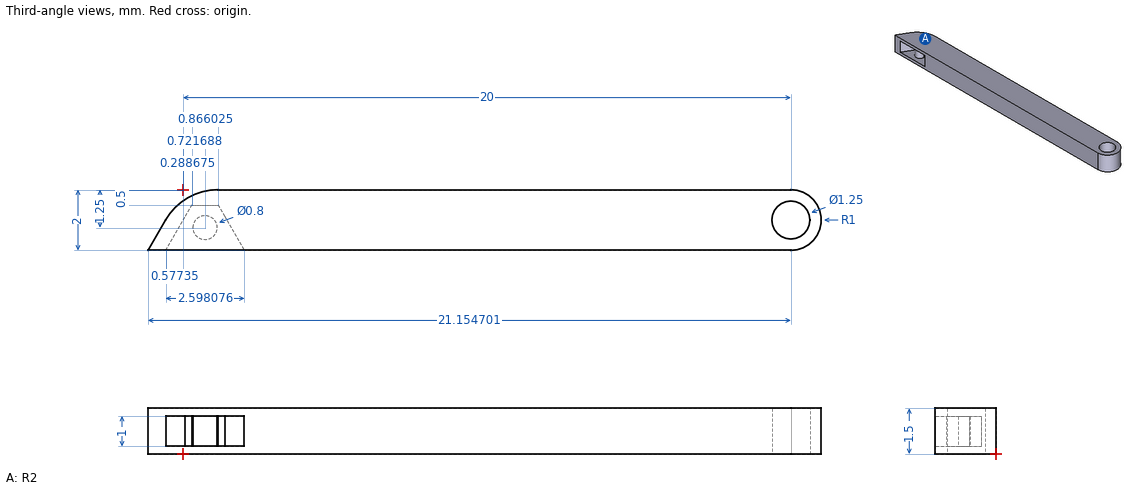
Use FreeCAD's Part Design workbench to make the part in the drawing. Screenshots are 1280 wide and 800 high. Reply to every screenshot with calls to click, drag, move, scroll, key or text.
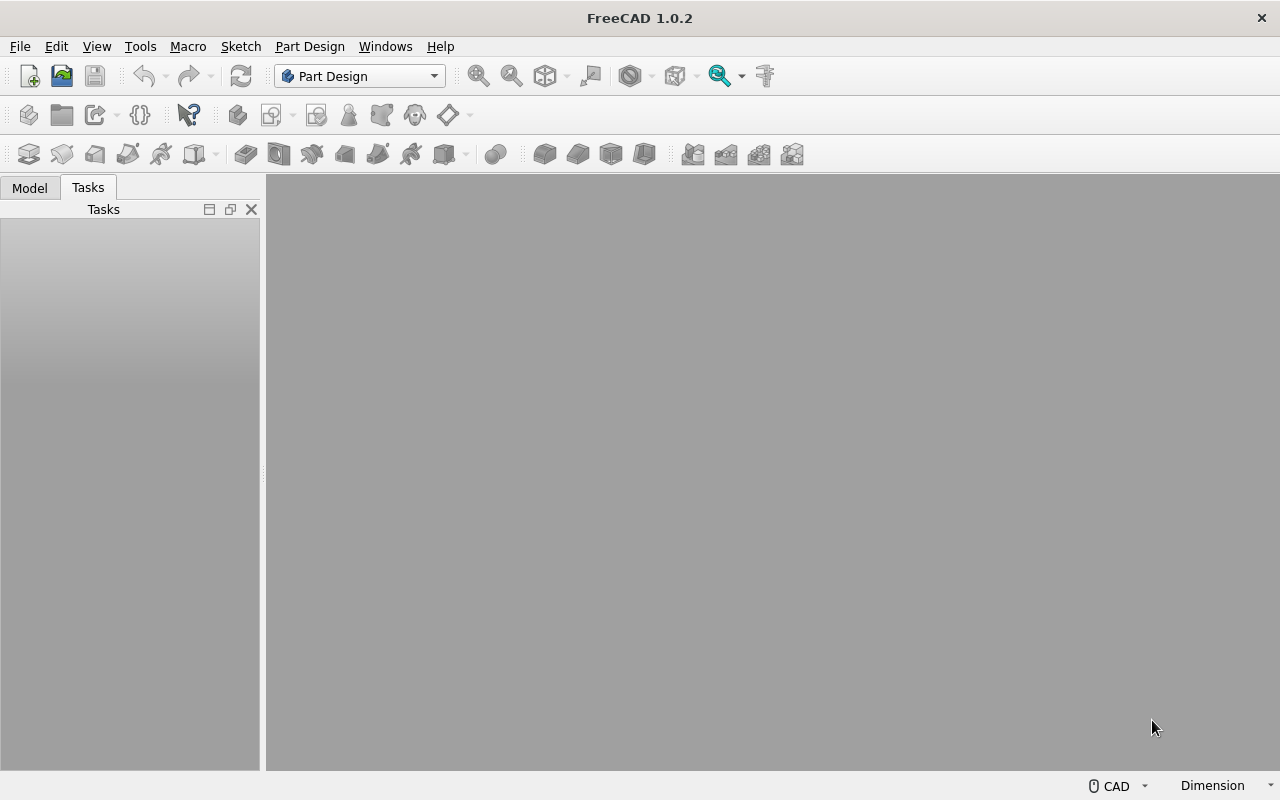
key(ctrl+n)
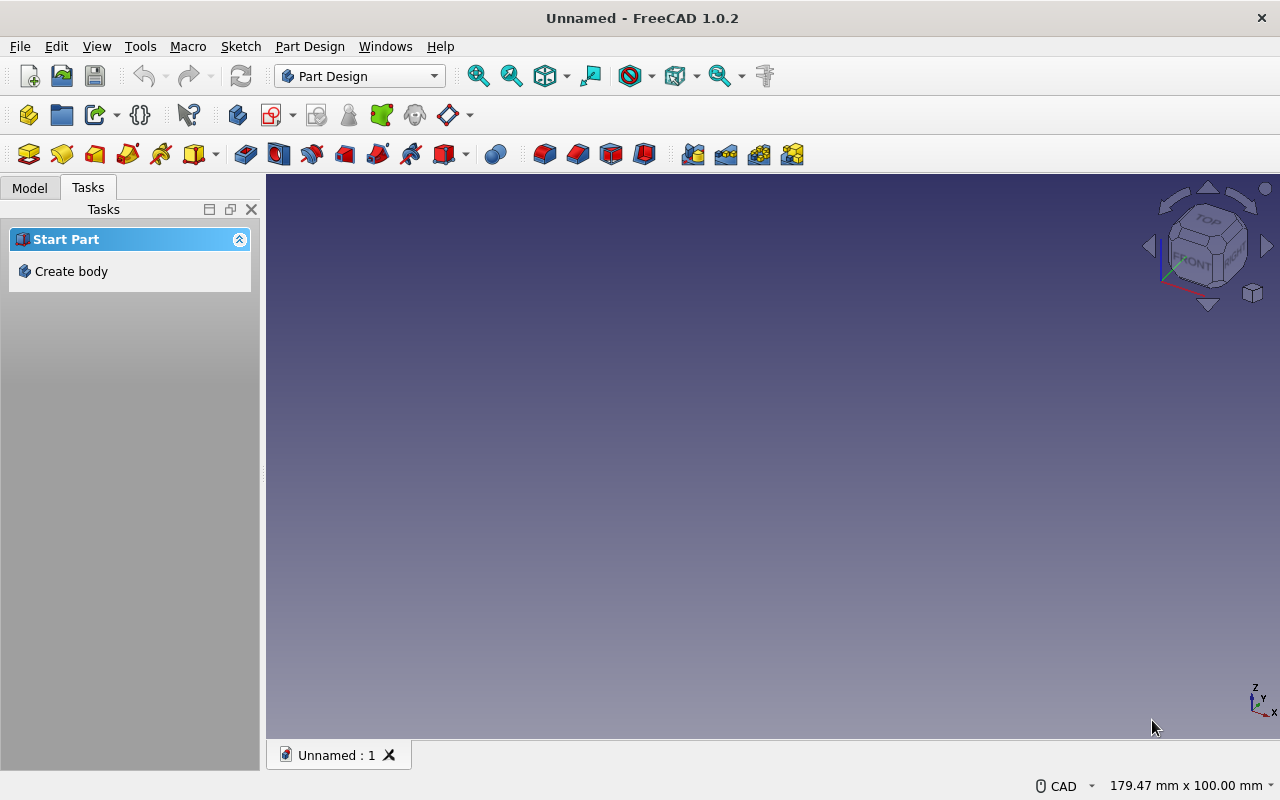
click(270, 116)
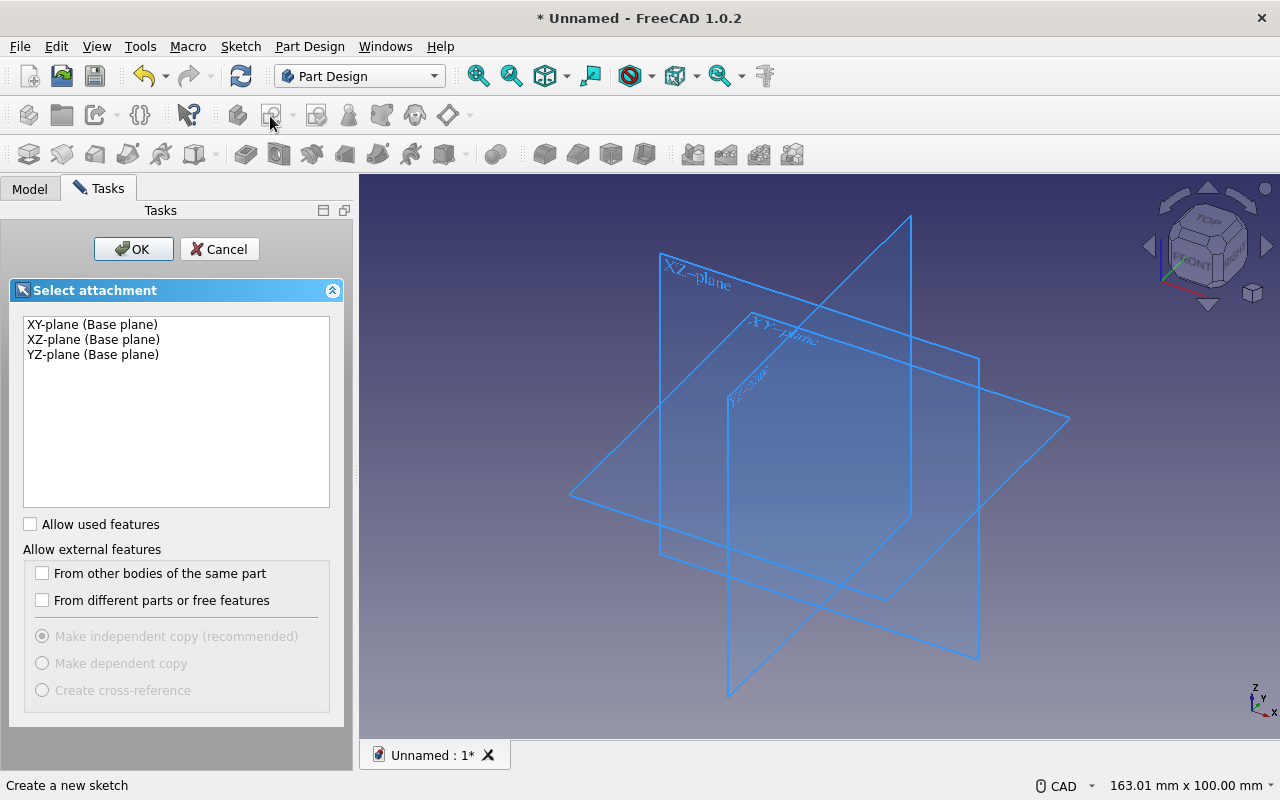
click(84, 324)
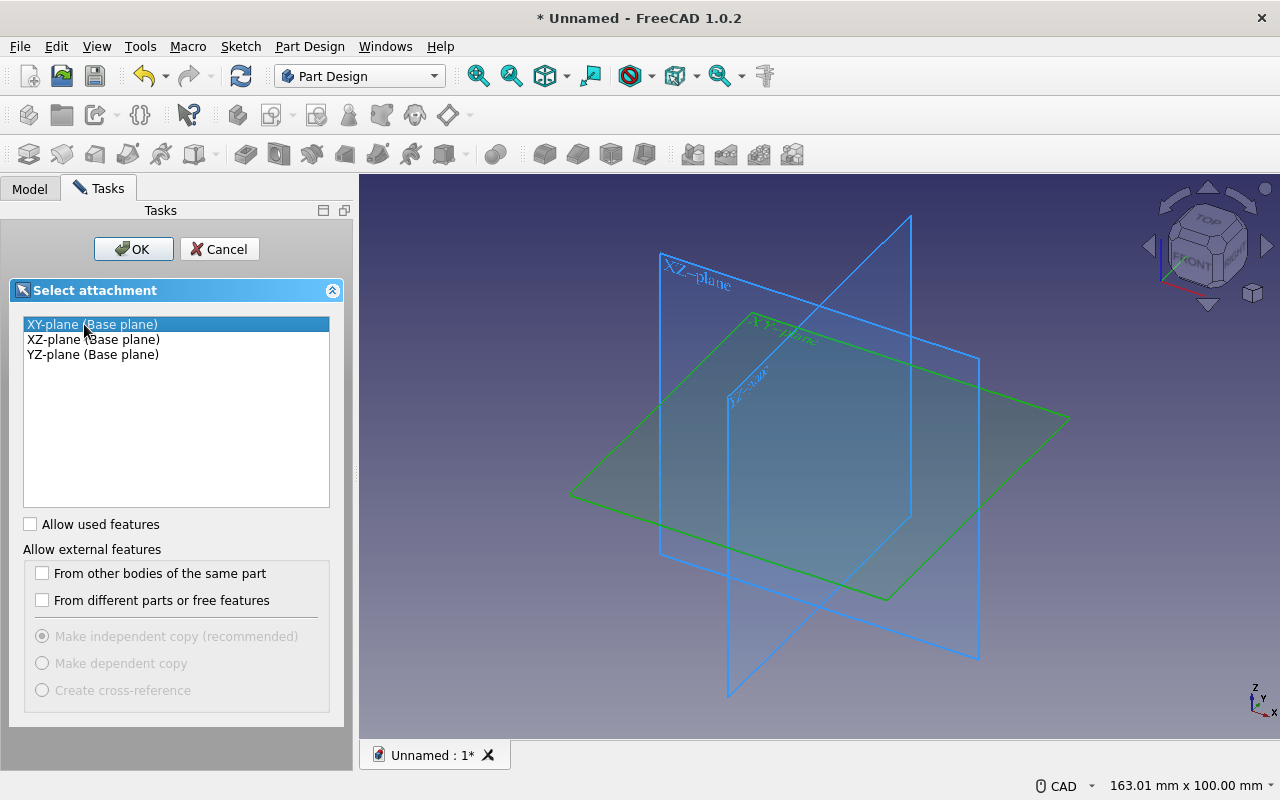
click(134, 249)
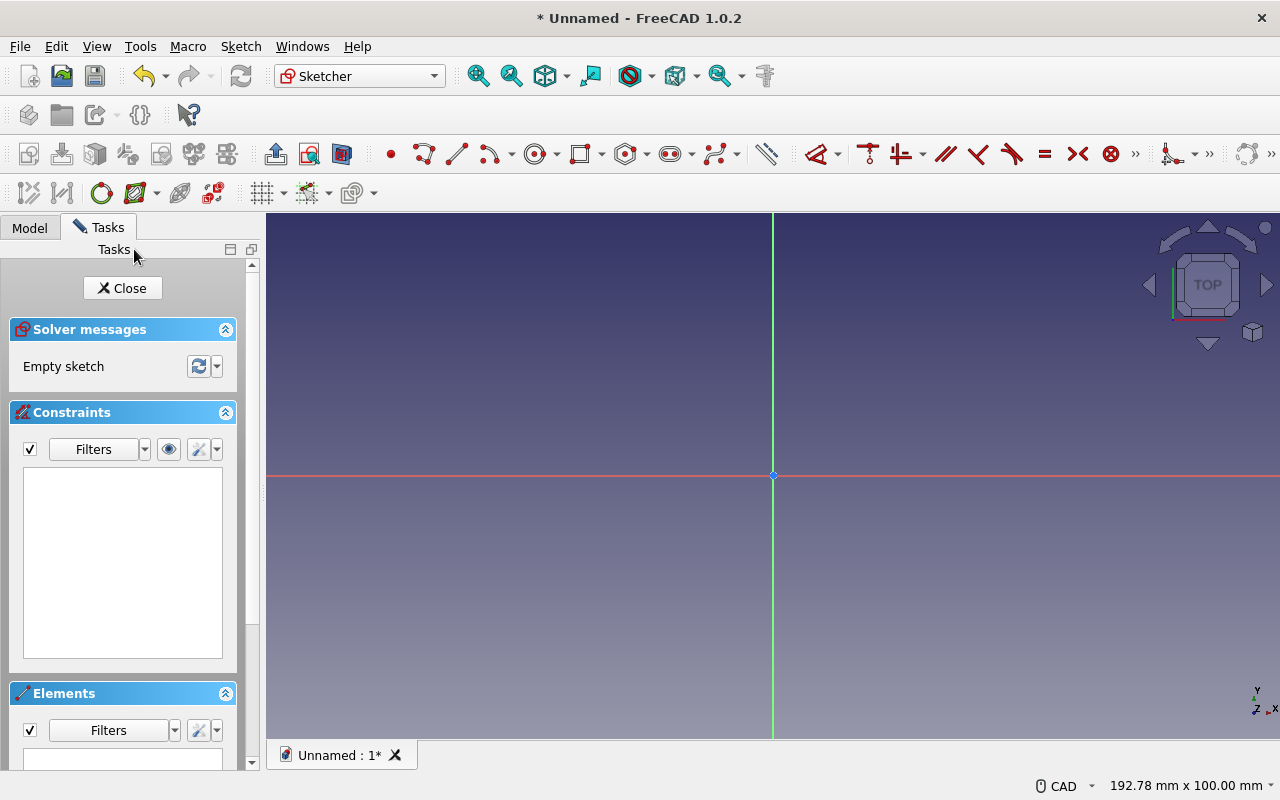
scroll(856, 483, up, 8)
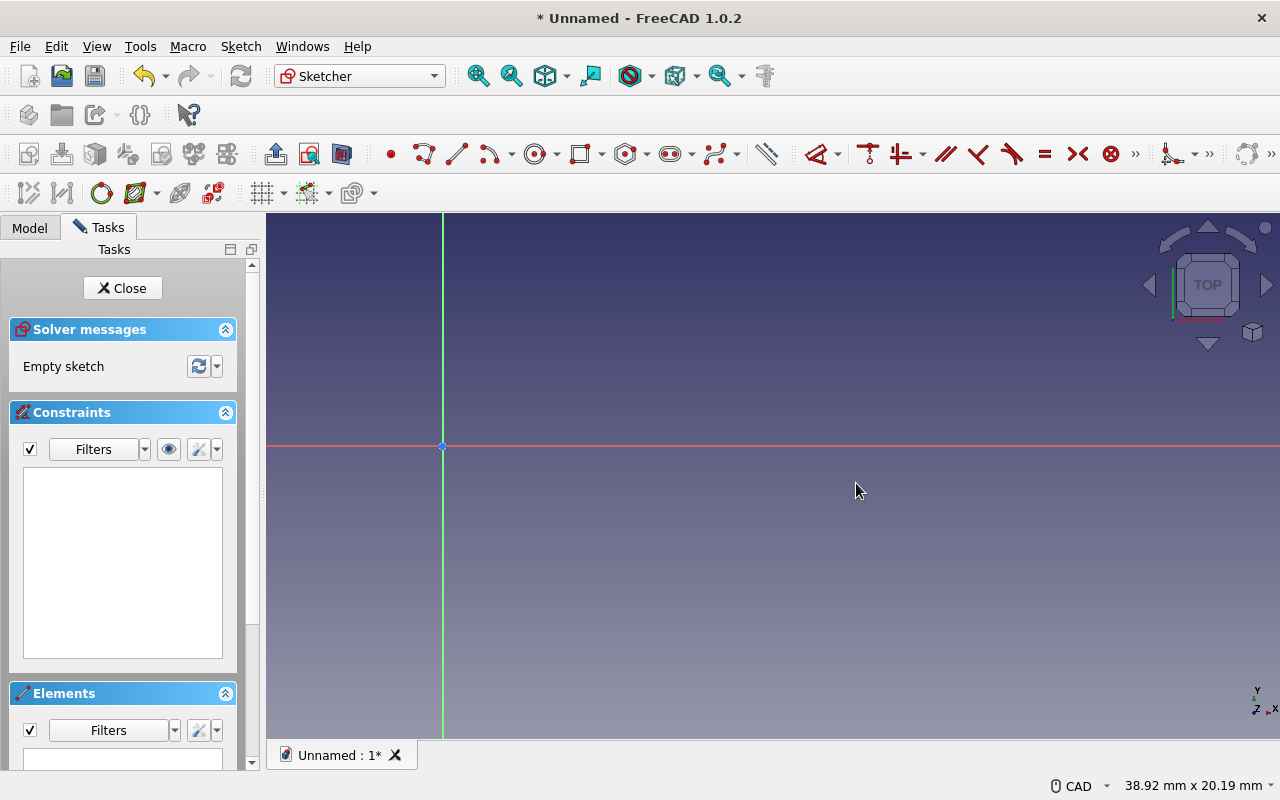
key(g)
key(m)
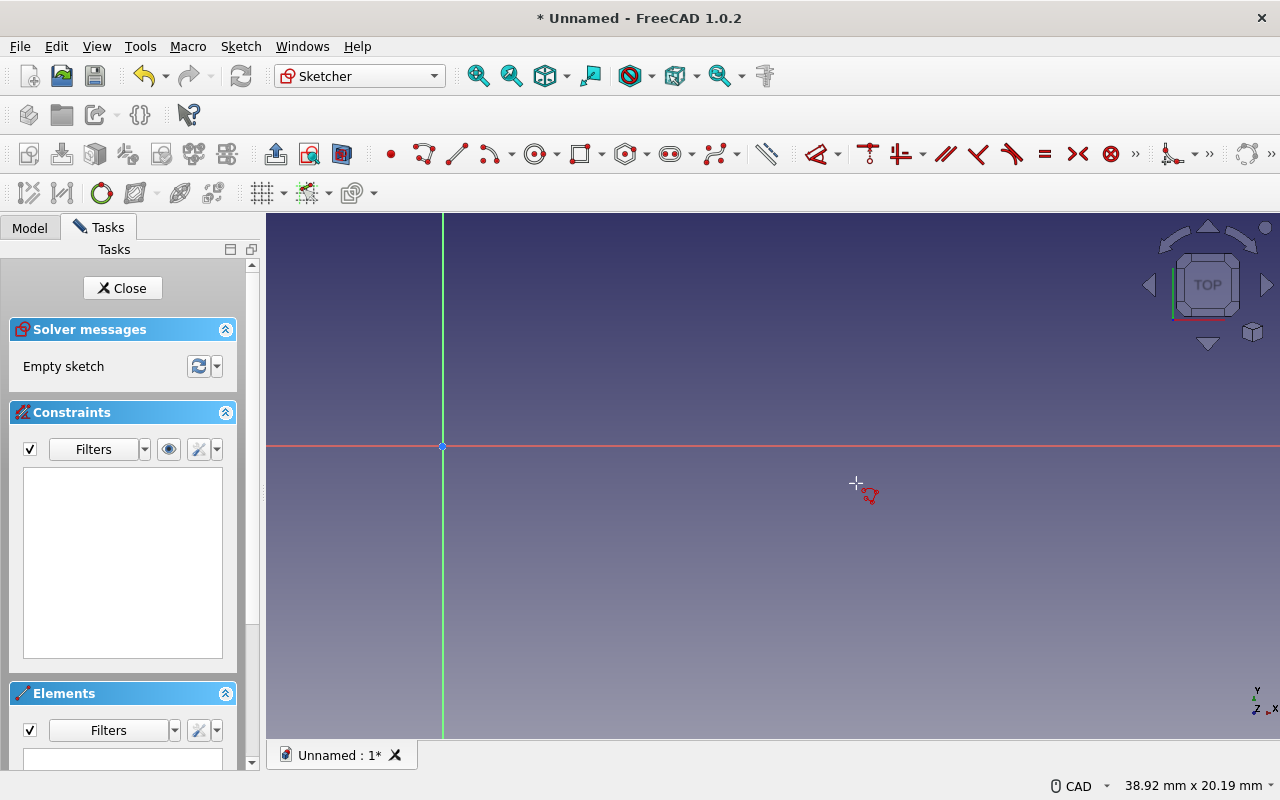
click(964, 446)
click(443, 446)
click(413, 498)
click(964, 498)
right_click(964, 498)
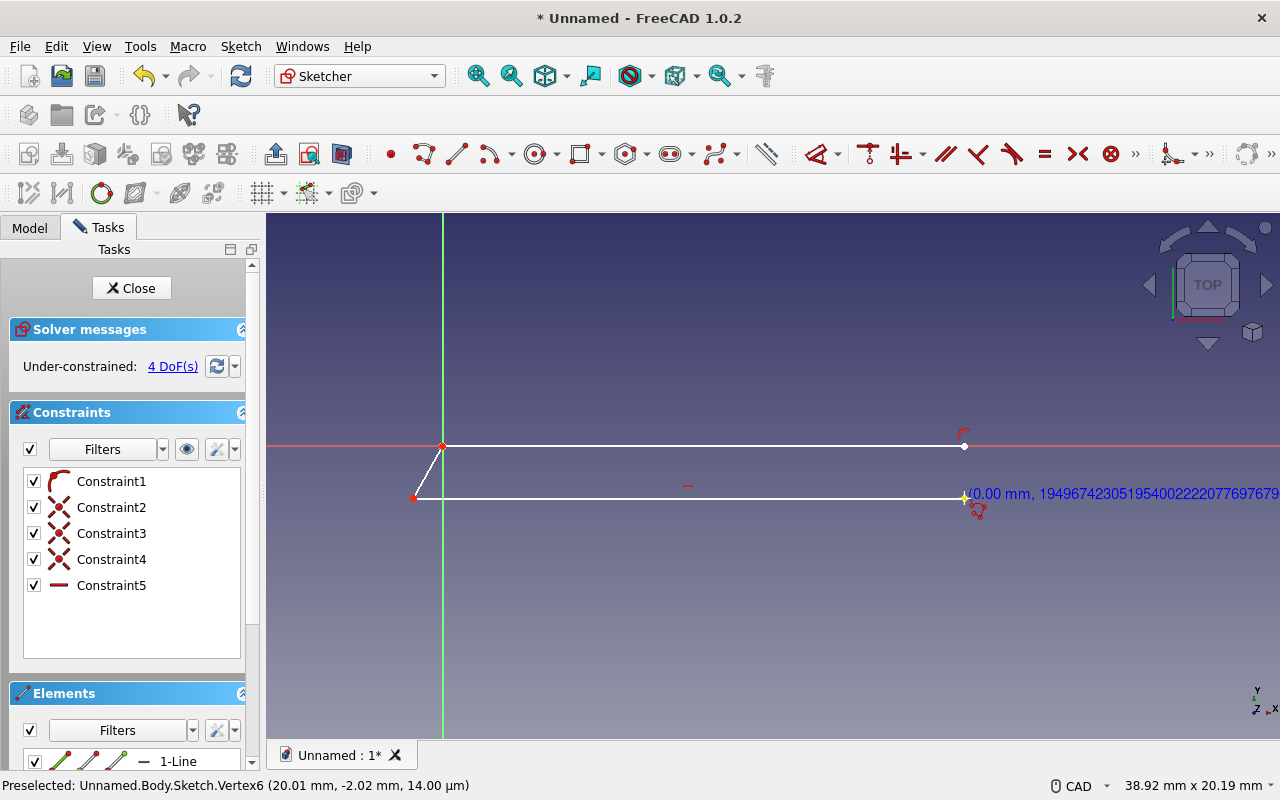
key(g)
key(3)
key(a)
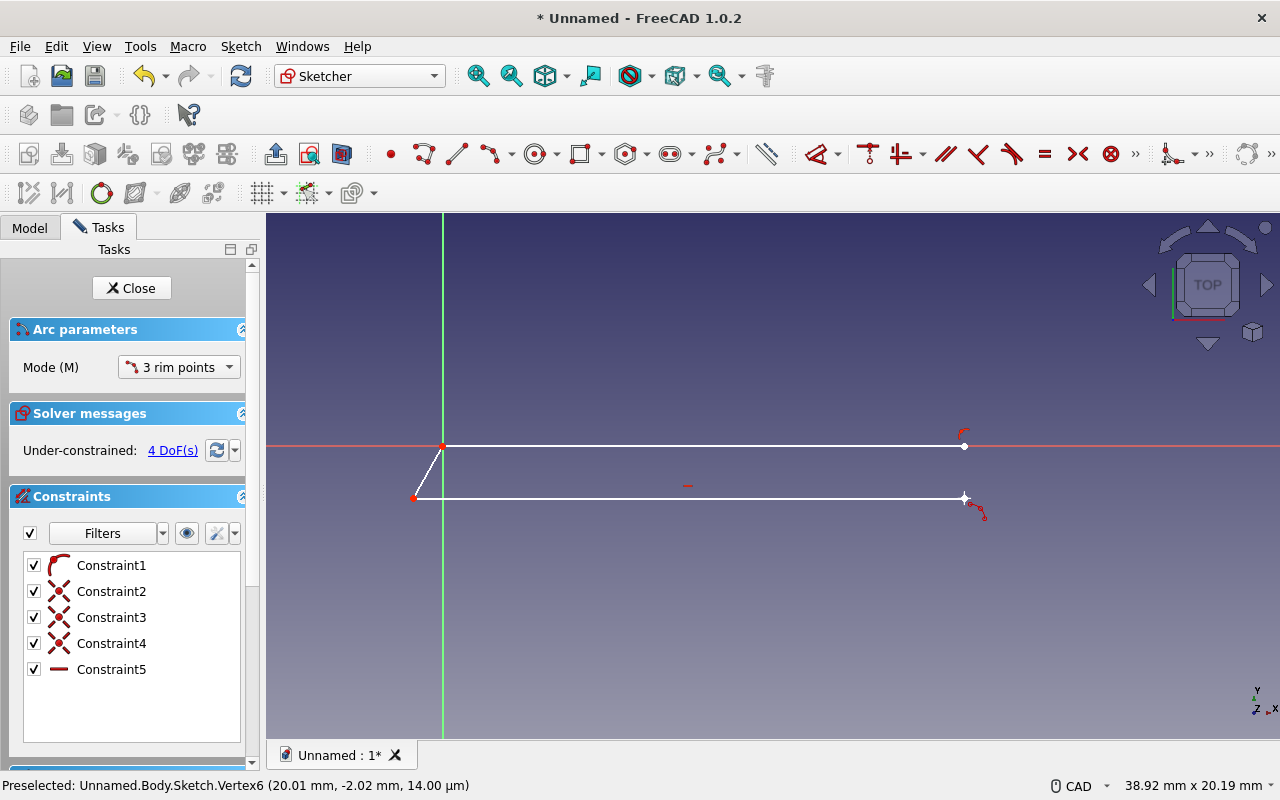
click(964, 499)
click(964, 446)
click(990, 472)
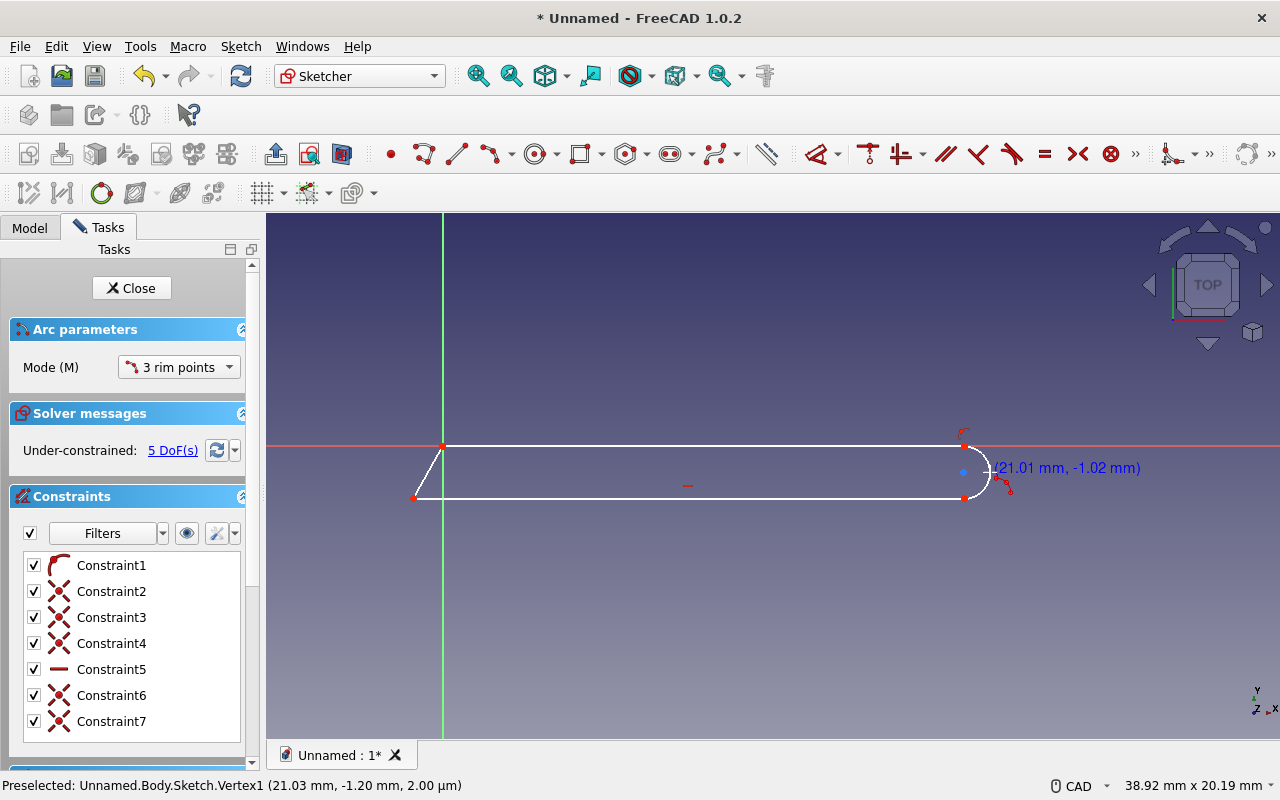
key(g)
key(c)